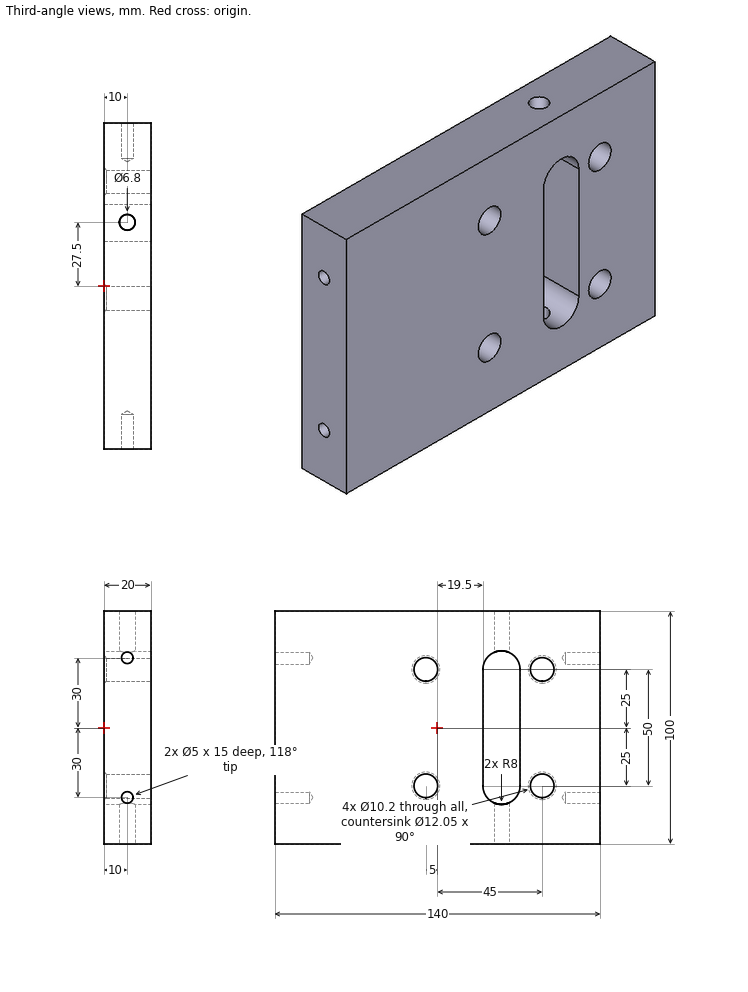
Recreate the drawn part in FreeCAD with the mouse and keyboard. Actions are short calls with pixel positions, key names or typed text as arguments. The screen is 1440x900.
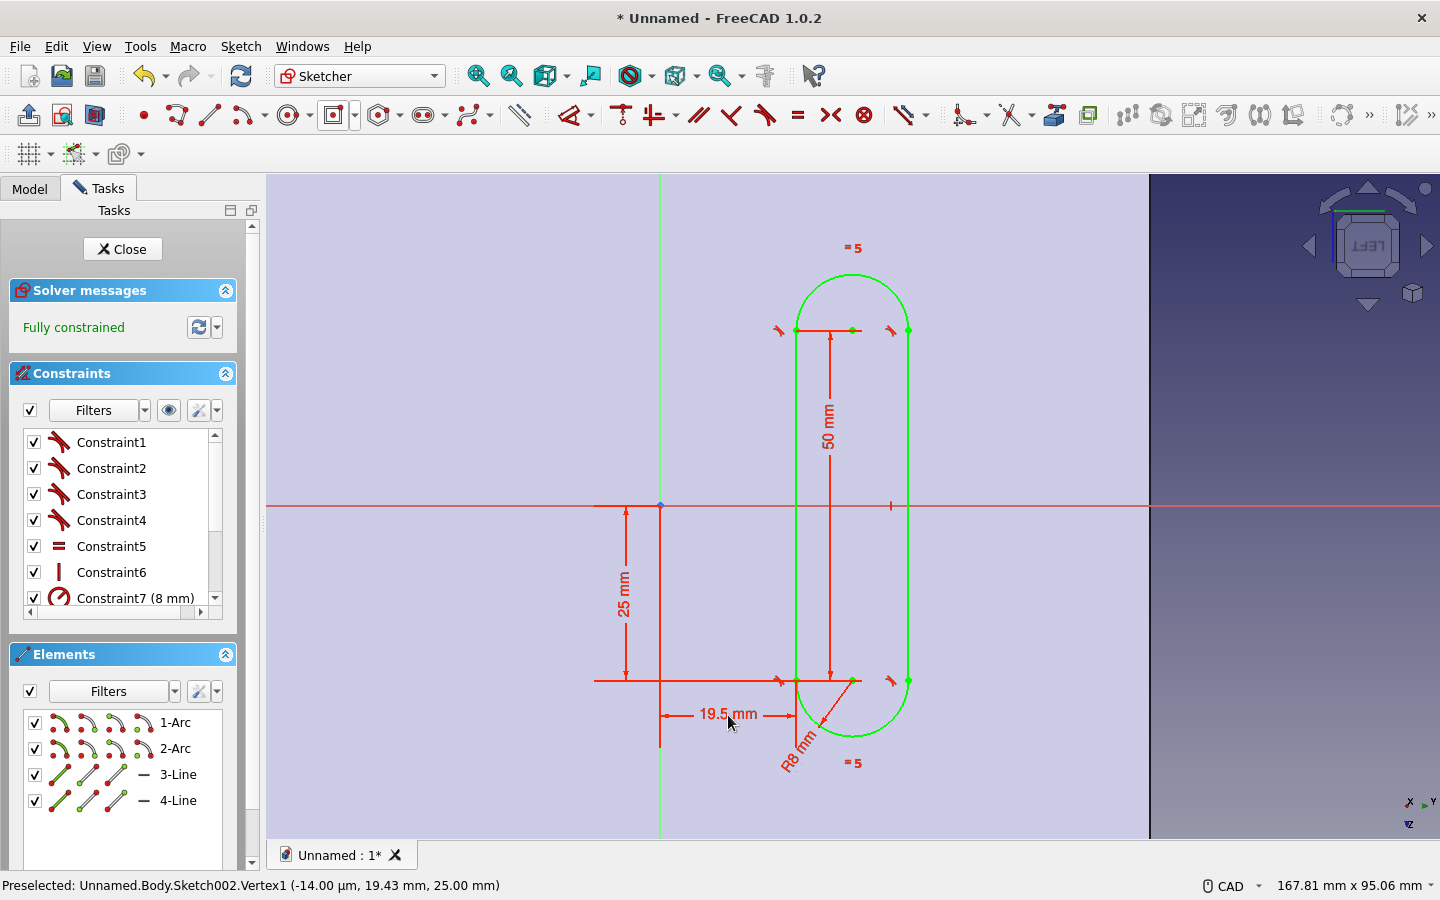
click(123, 249)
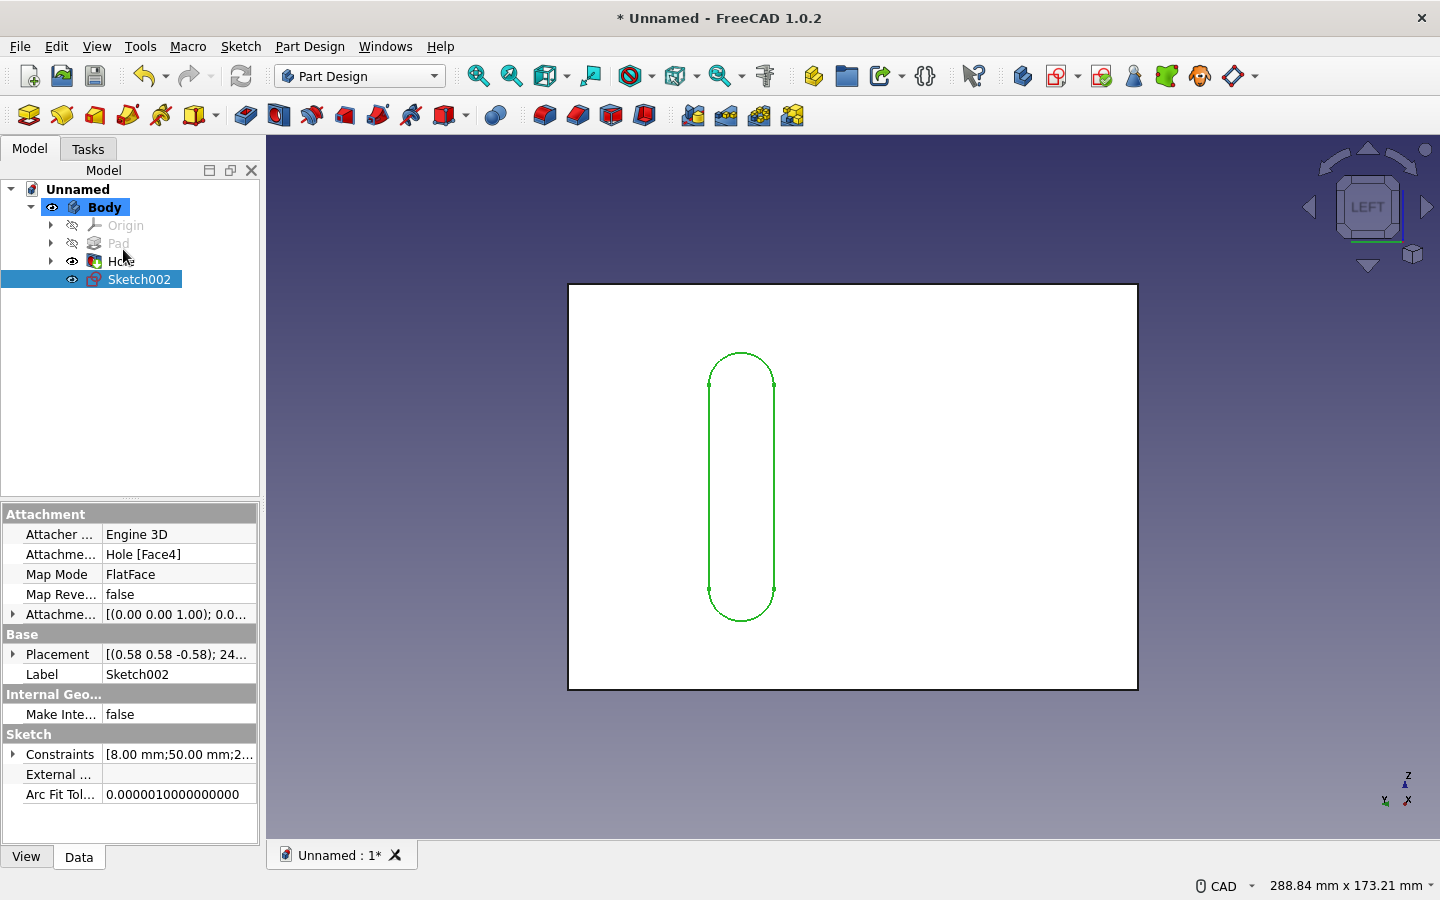
click(246, 116)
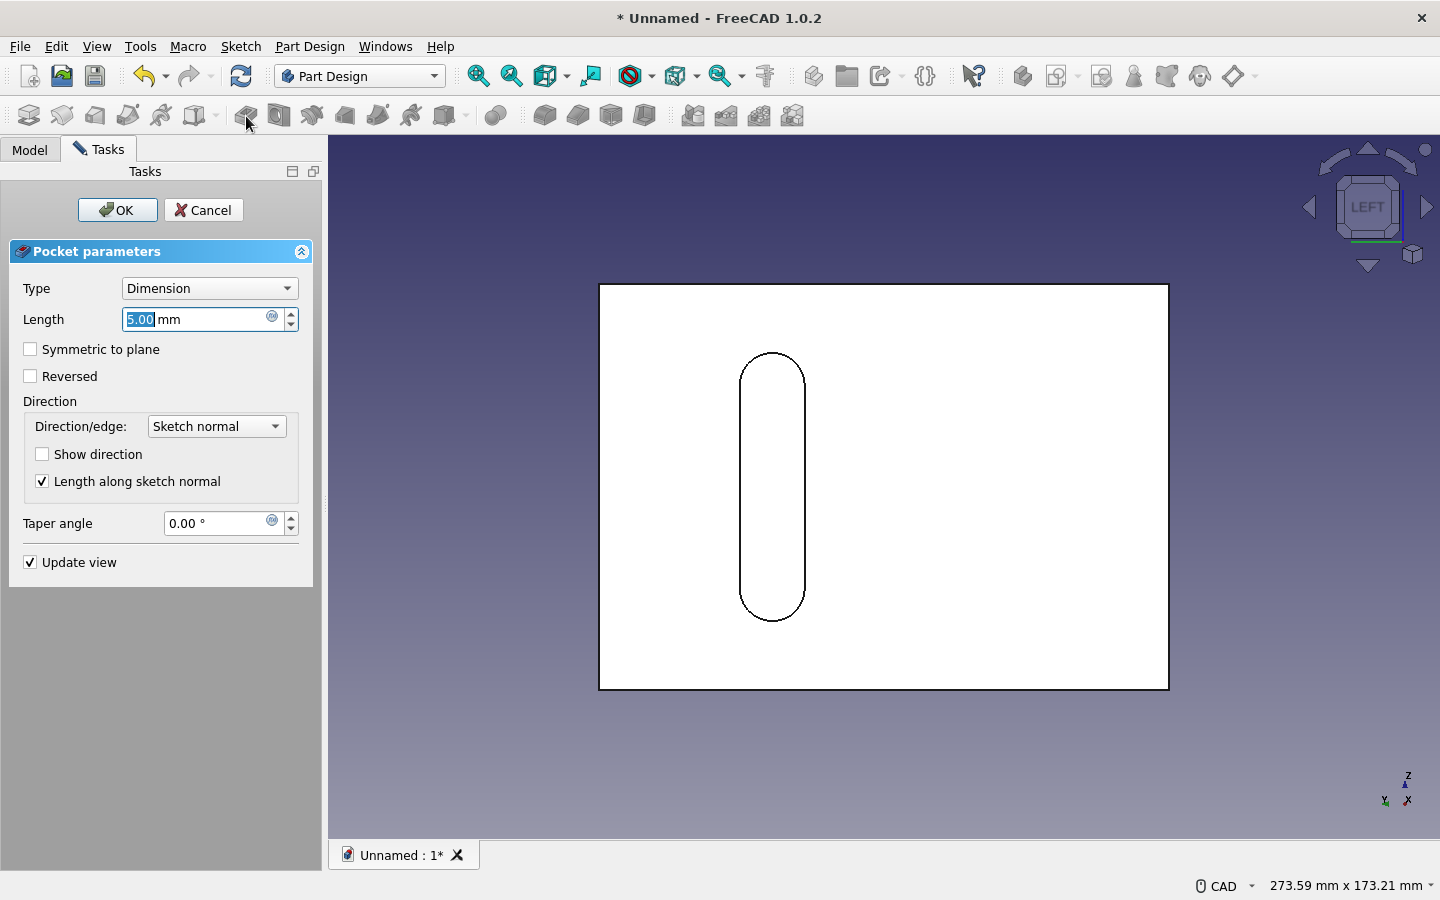
click(210, 288)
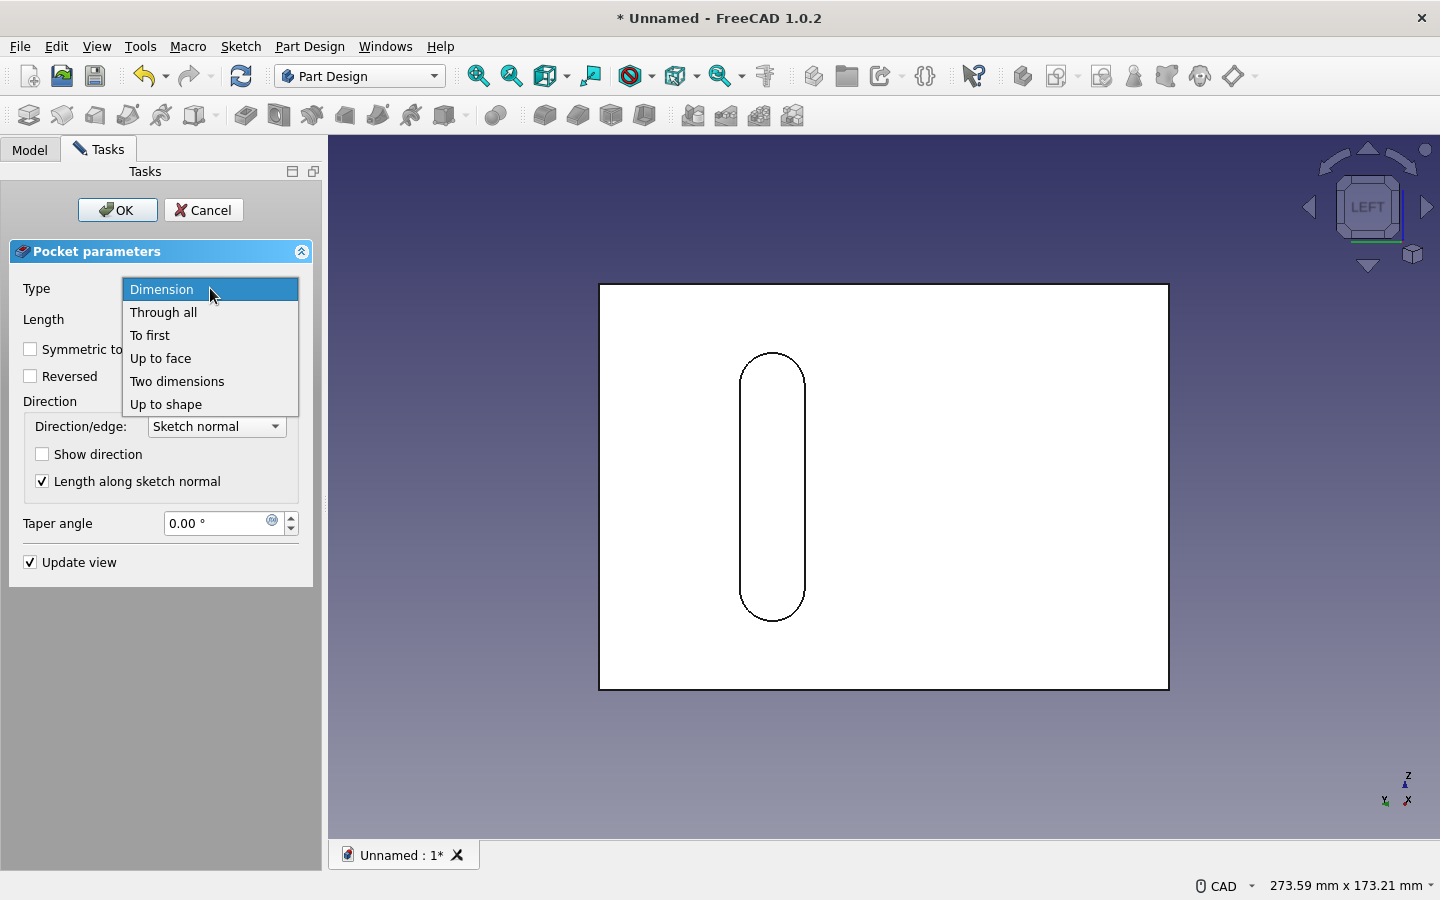
click(208, 312)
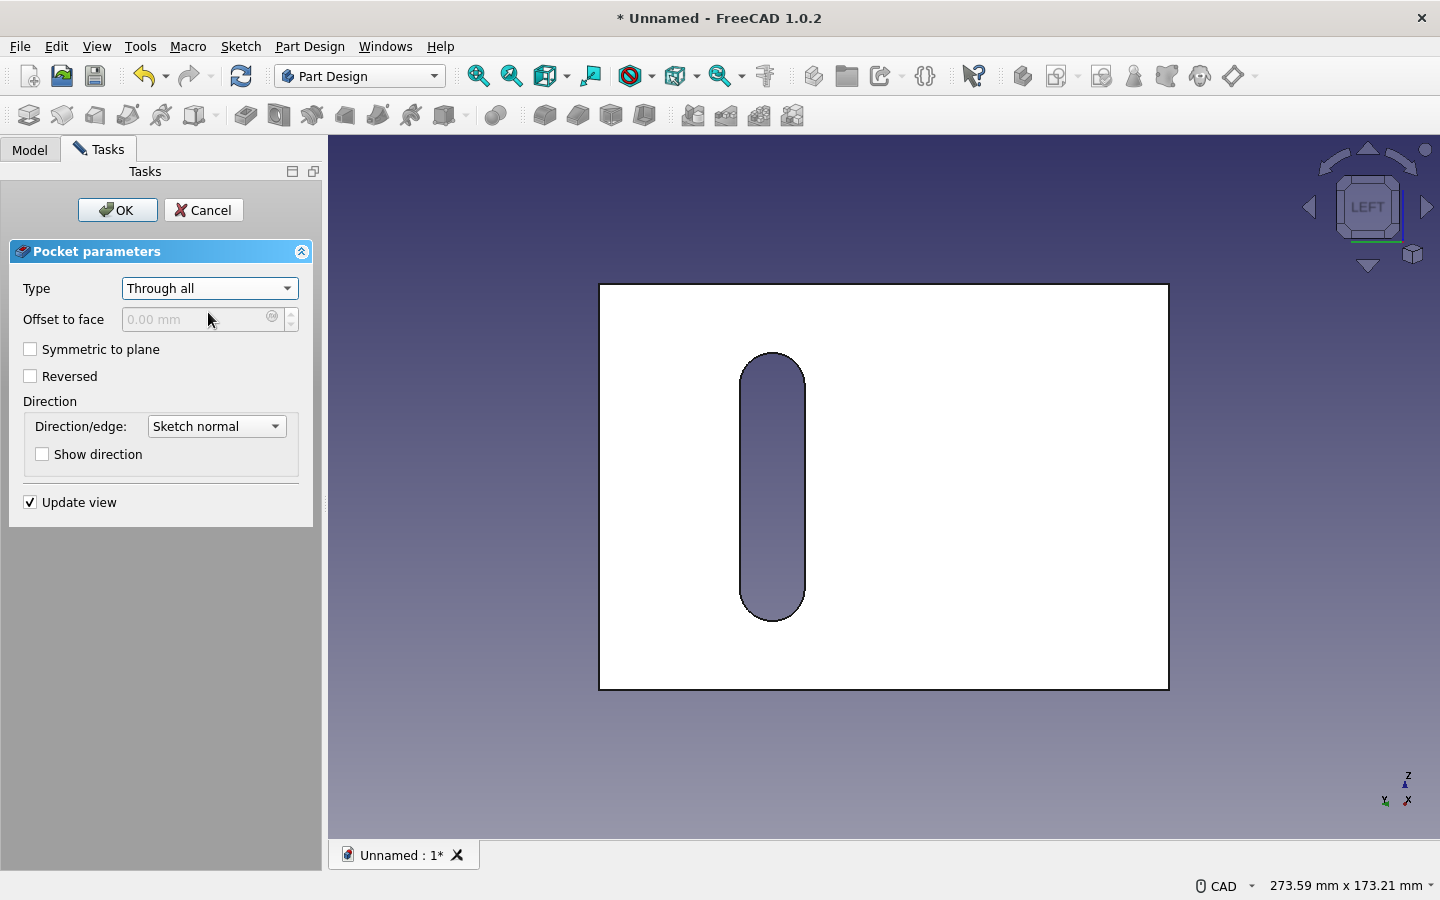
click(118, 210)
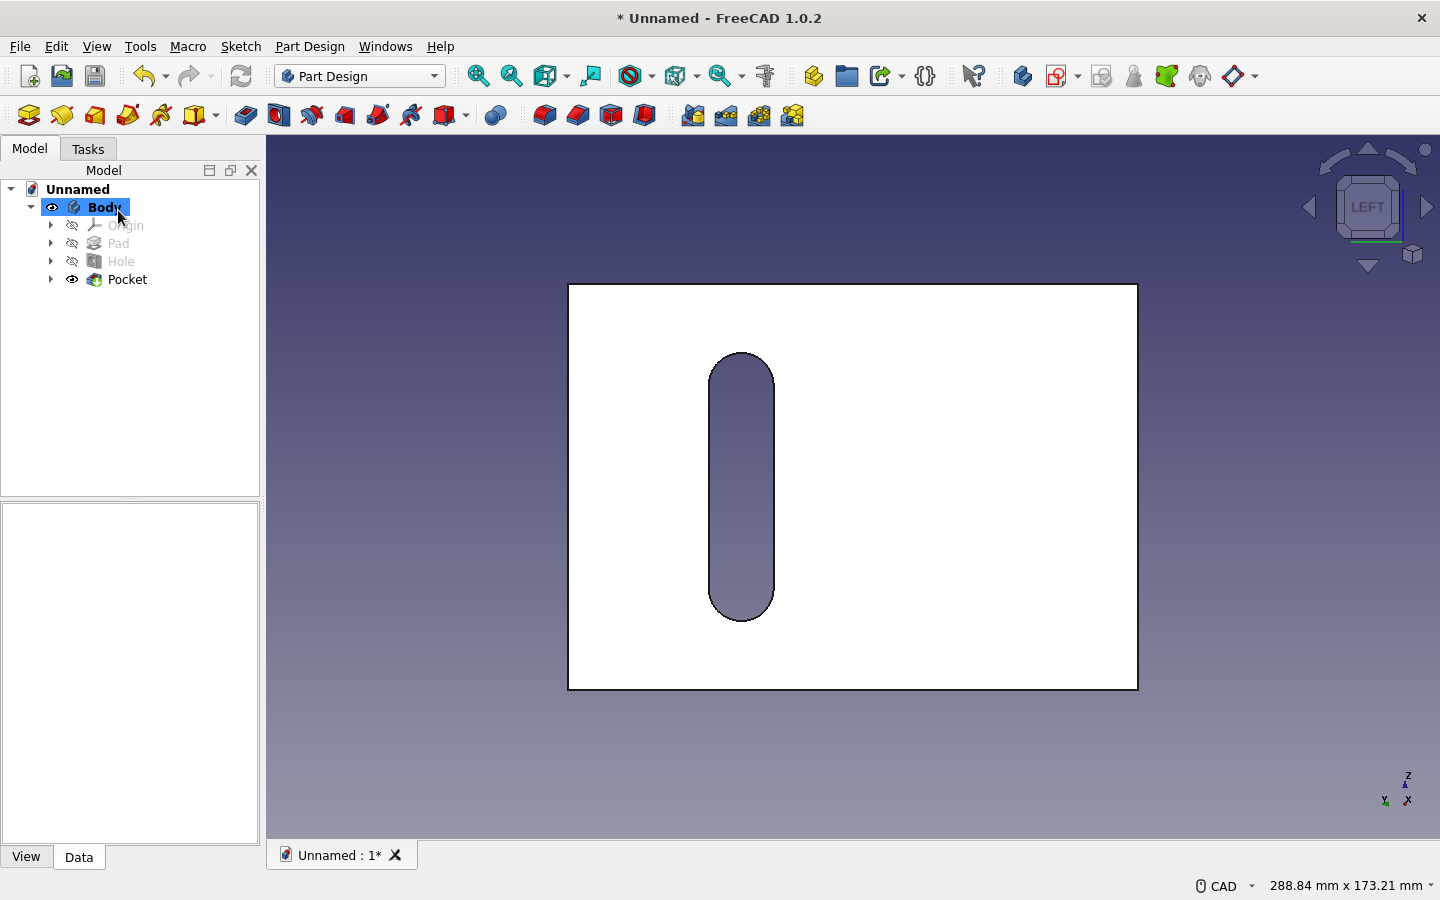
key(0)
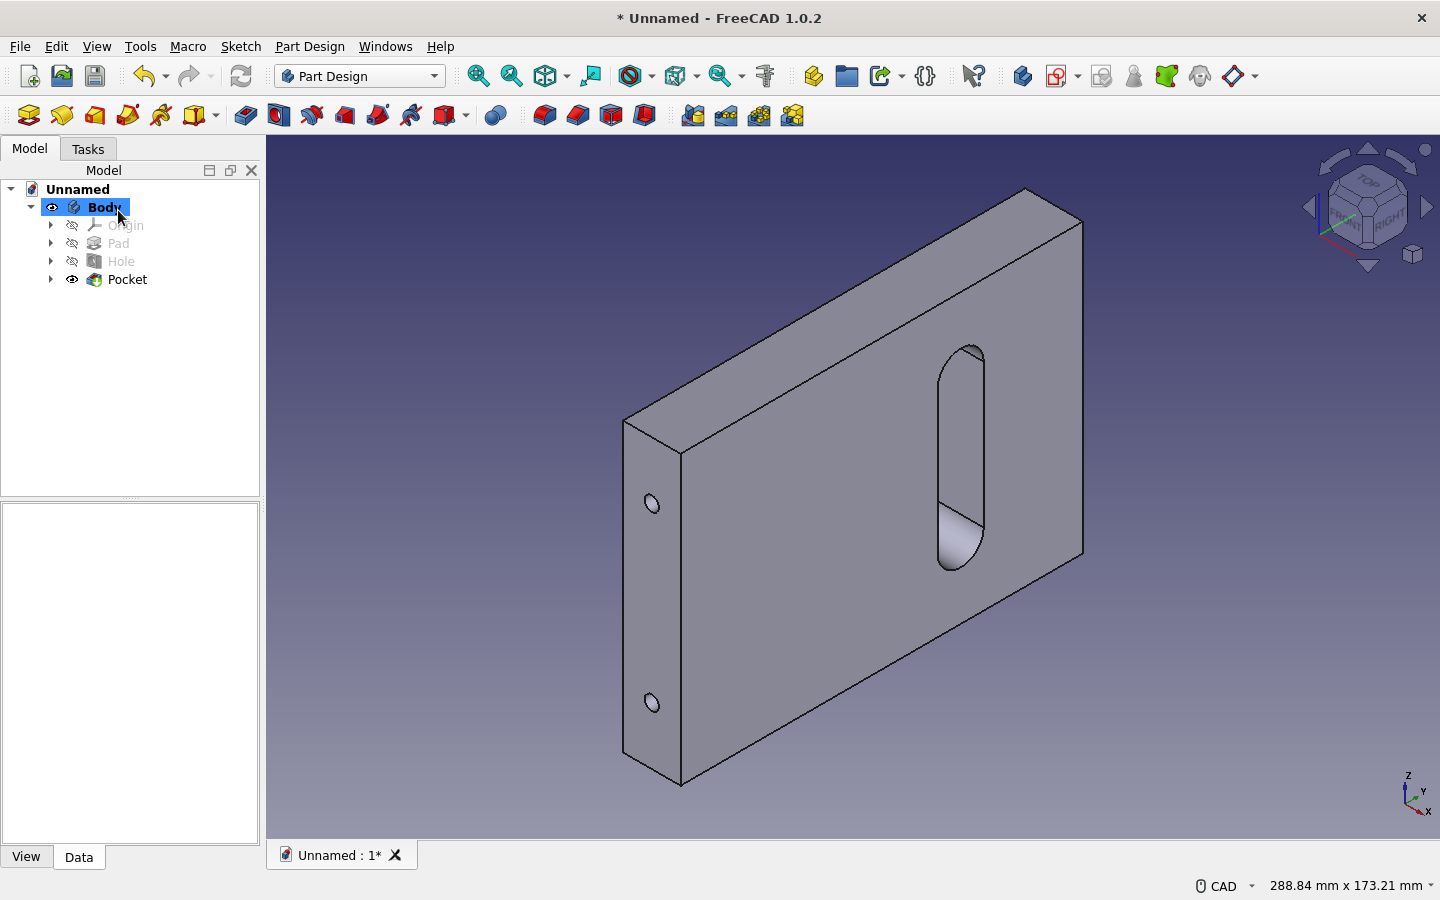
click(1025, 221)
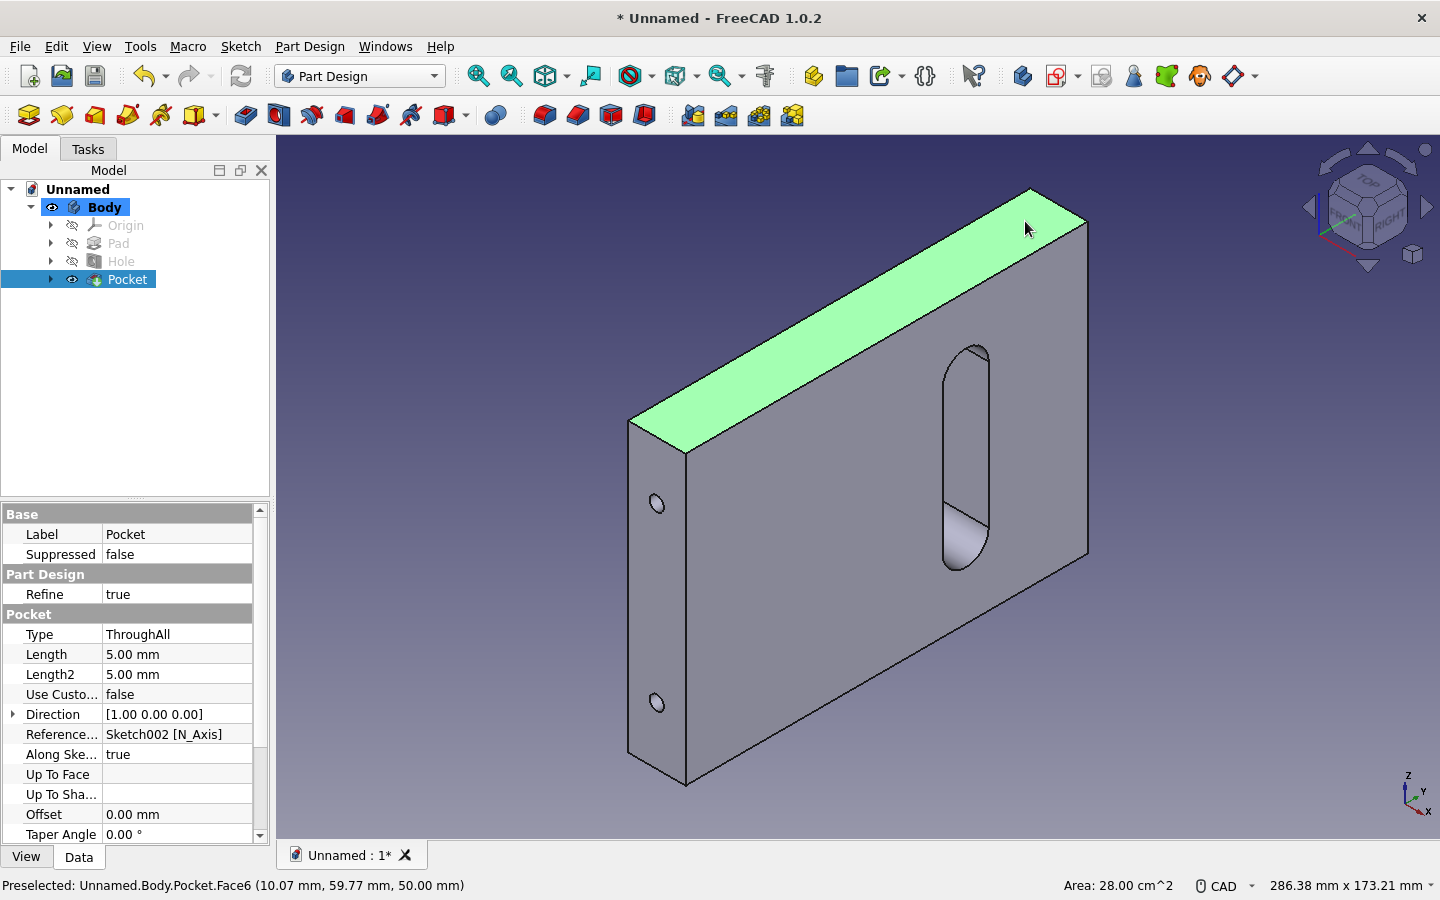
click(1056, 76)